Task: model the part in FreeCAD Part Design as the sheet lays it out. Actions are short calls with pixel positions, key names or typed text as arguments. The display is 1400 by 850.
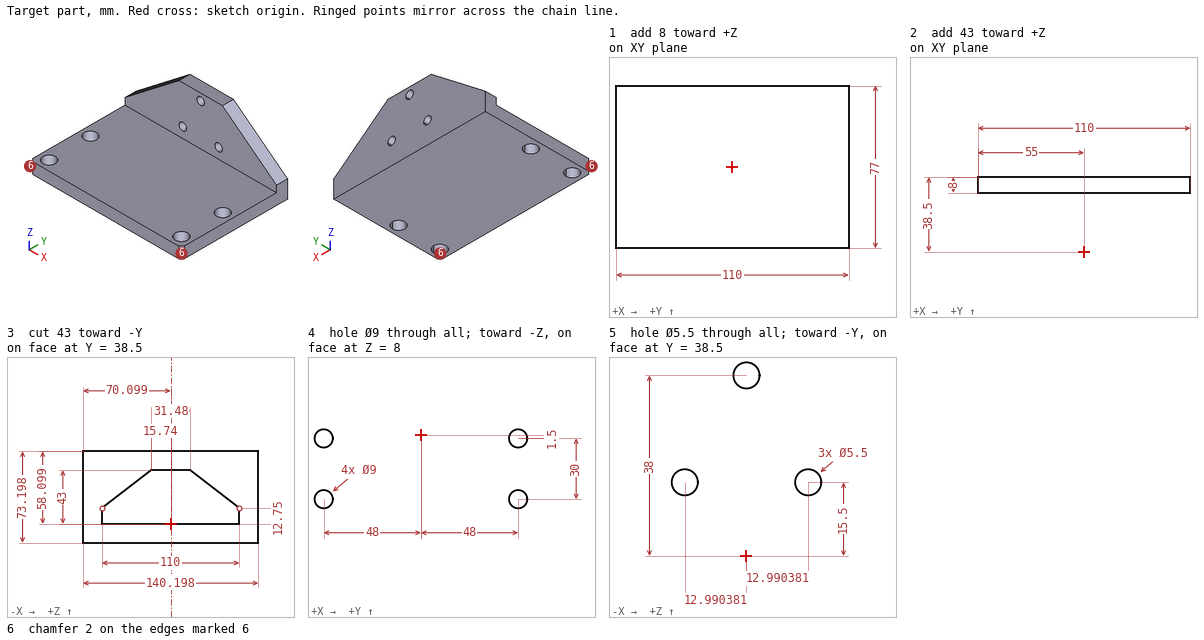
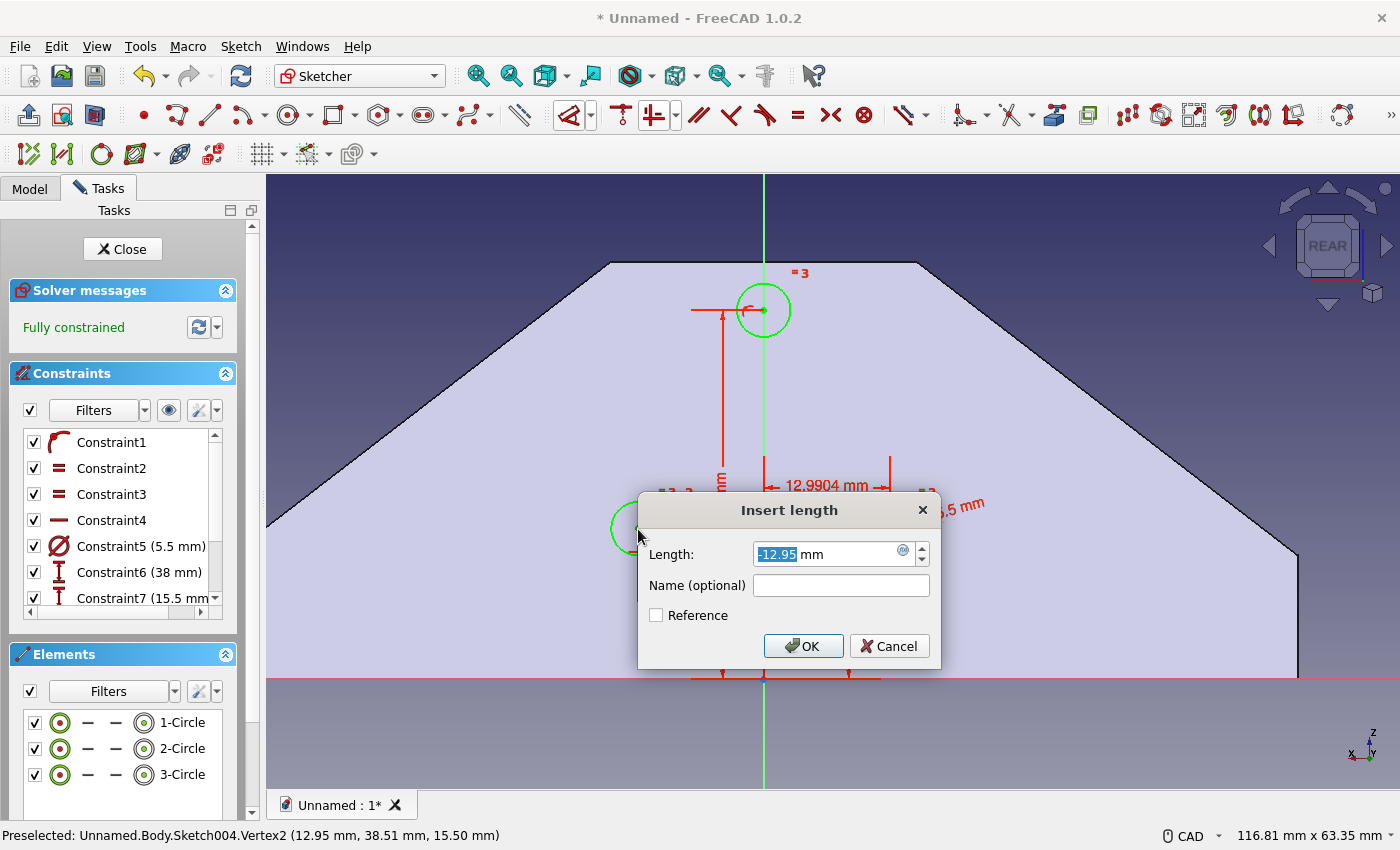
text(-12.990381)
key(Return)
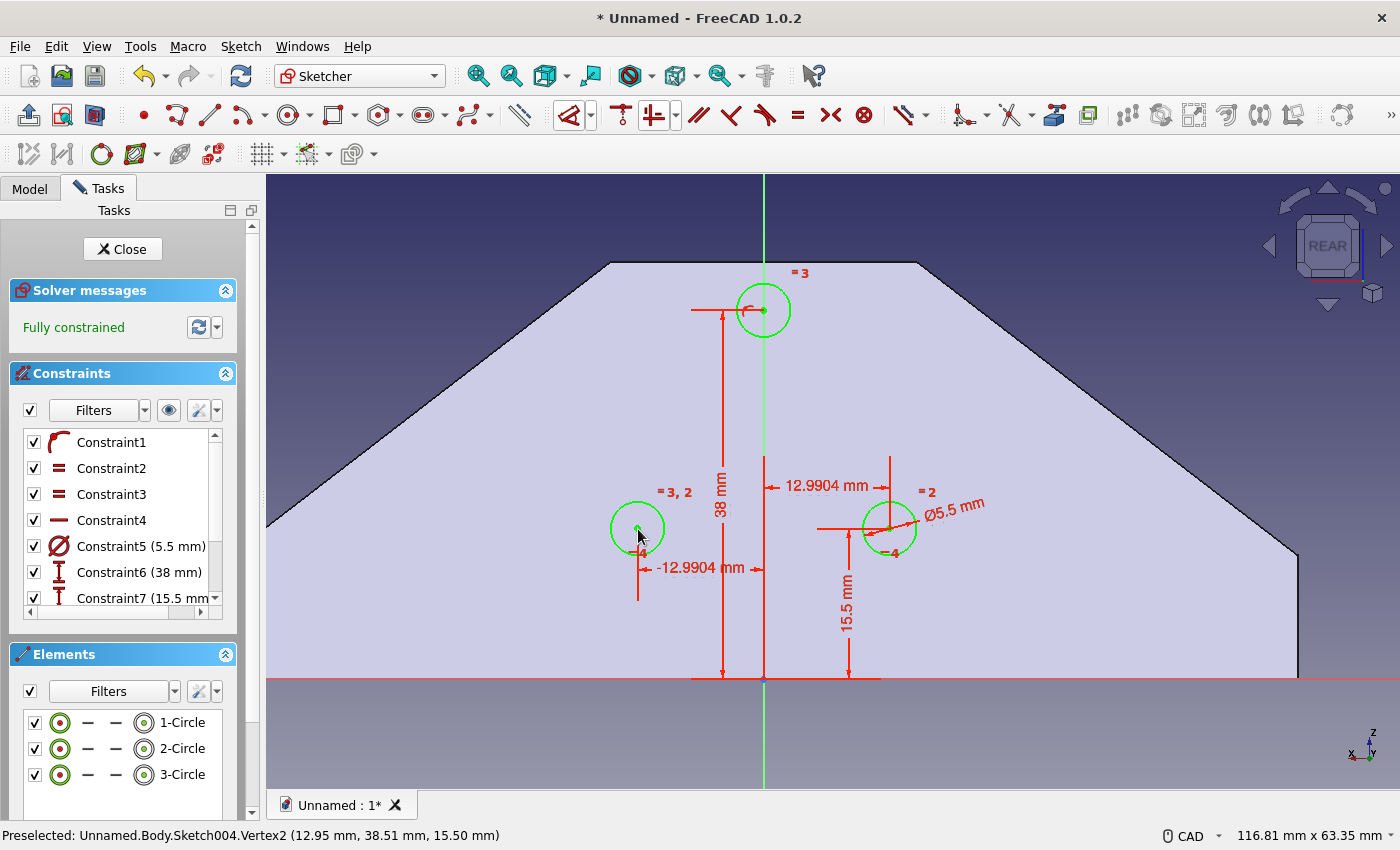
click(123, 249)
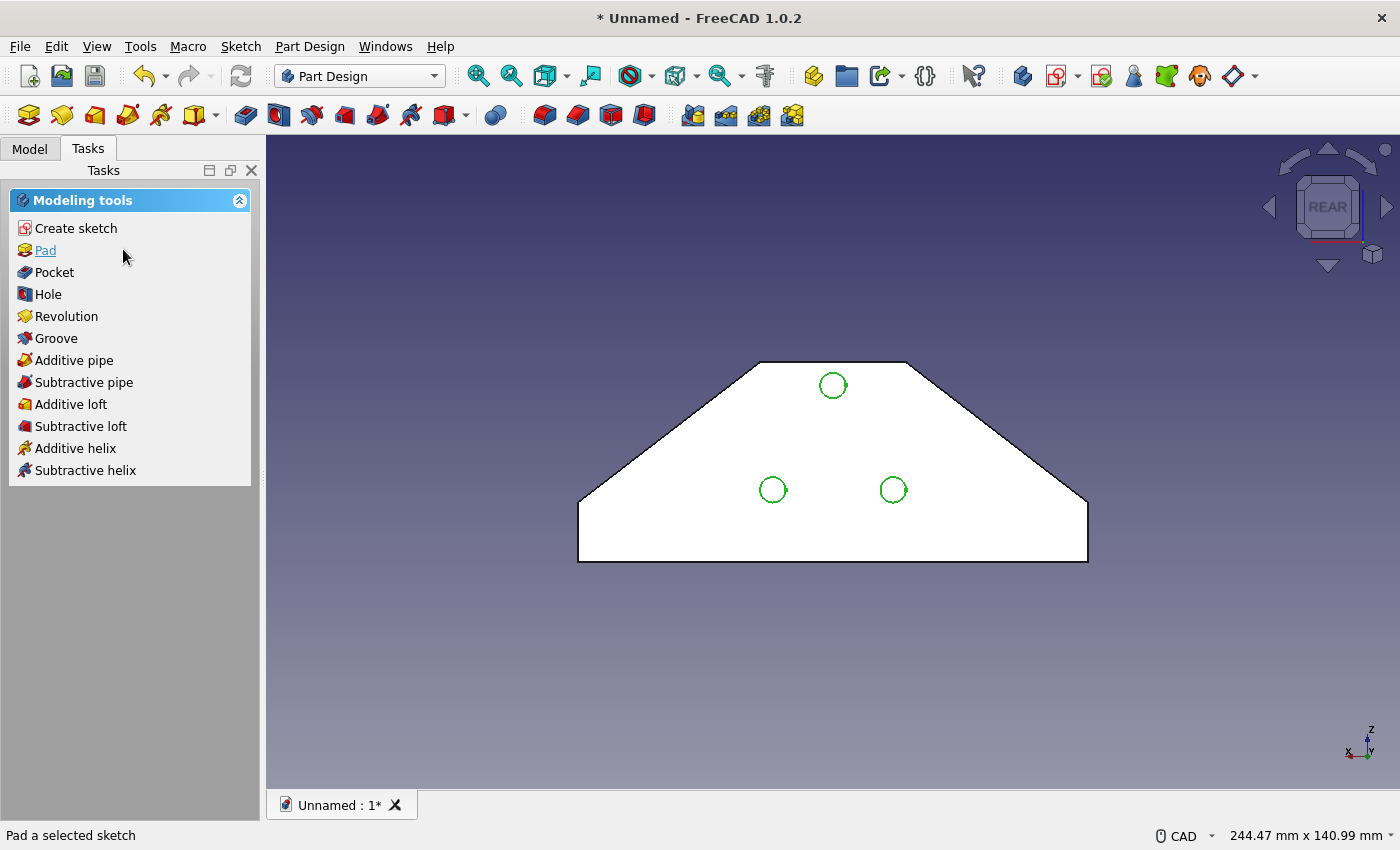
click(279, 116)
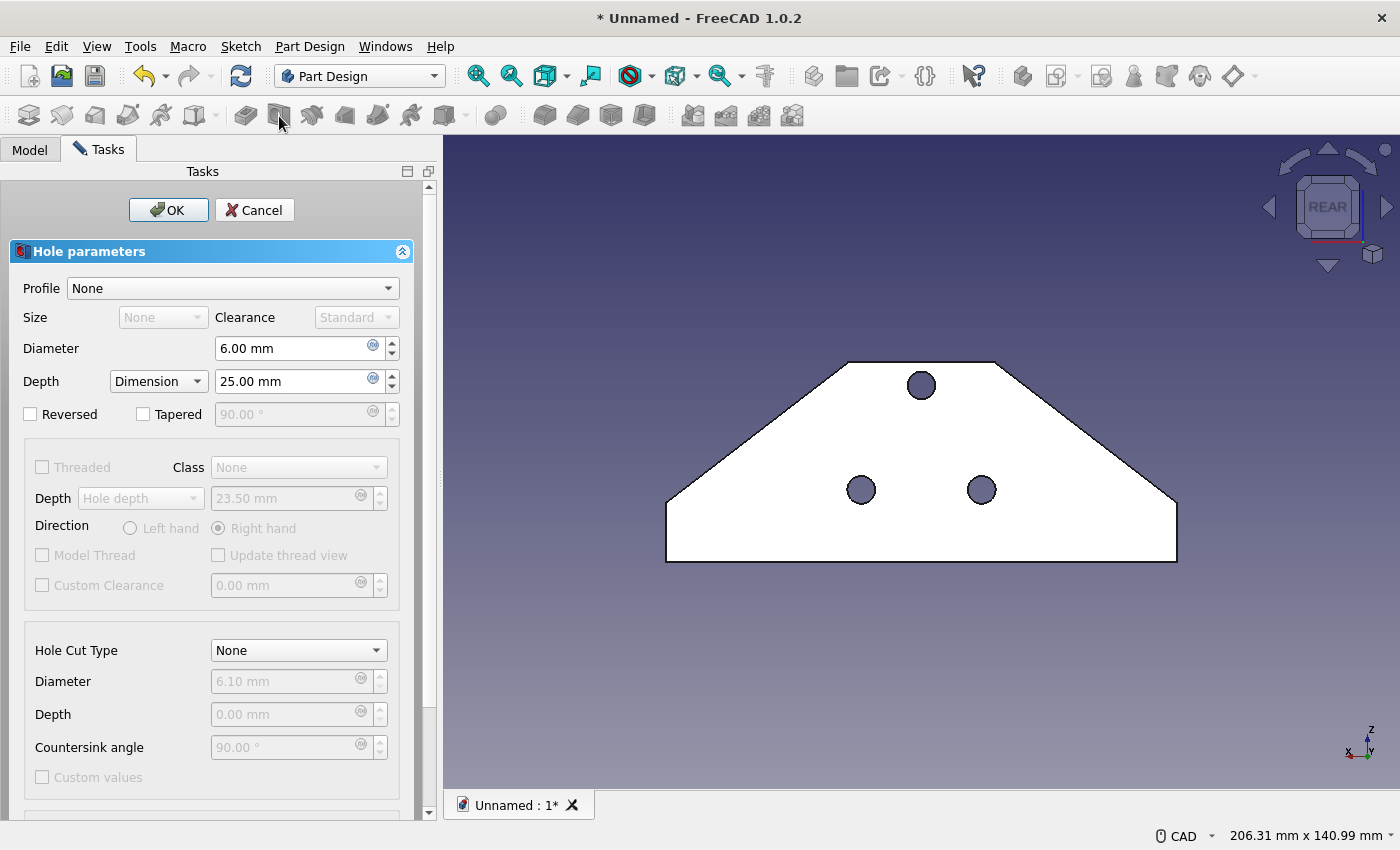
triple_click(300, 348)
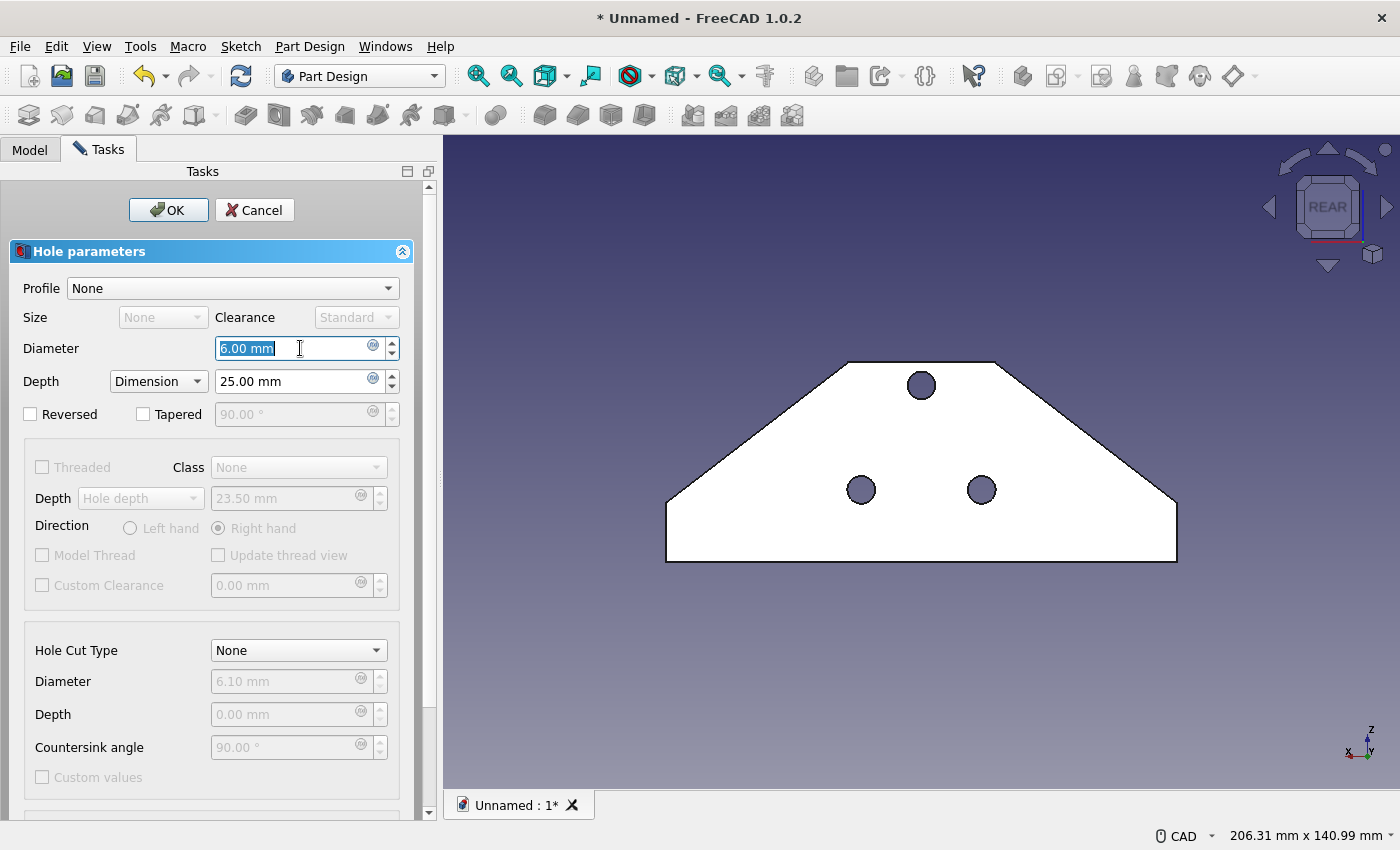
text(5.5)
key(Tab)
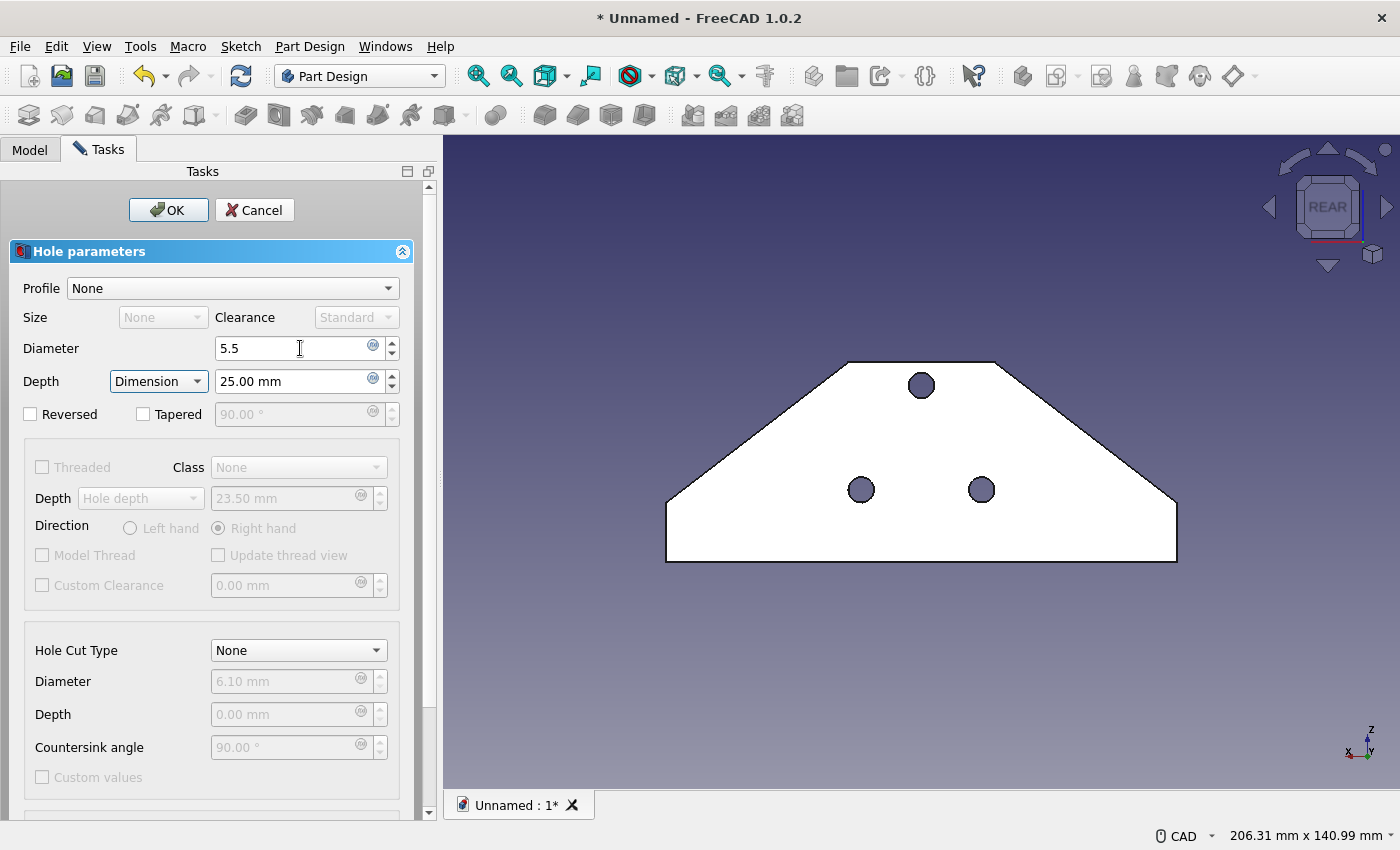
click(160, 382)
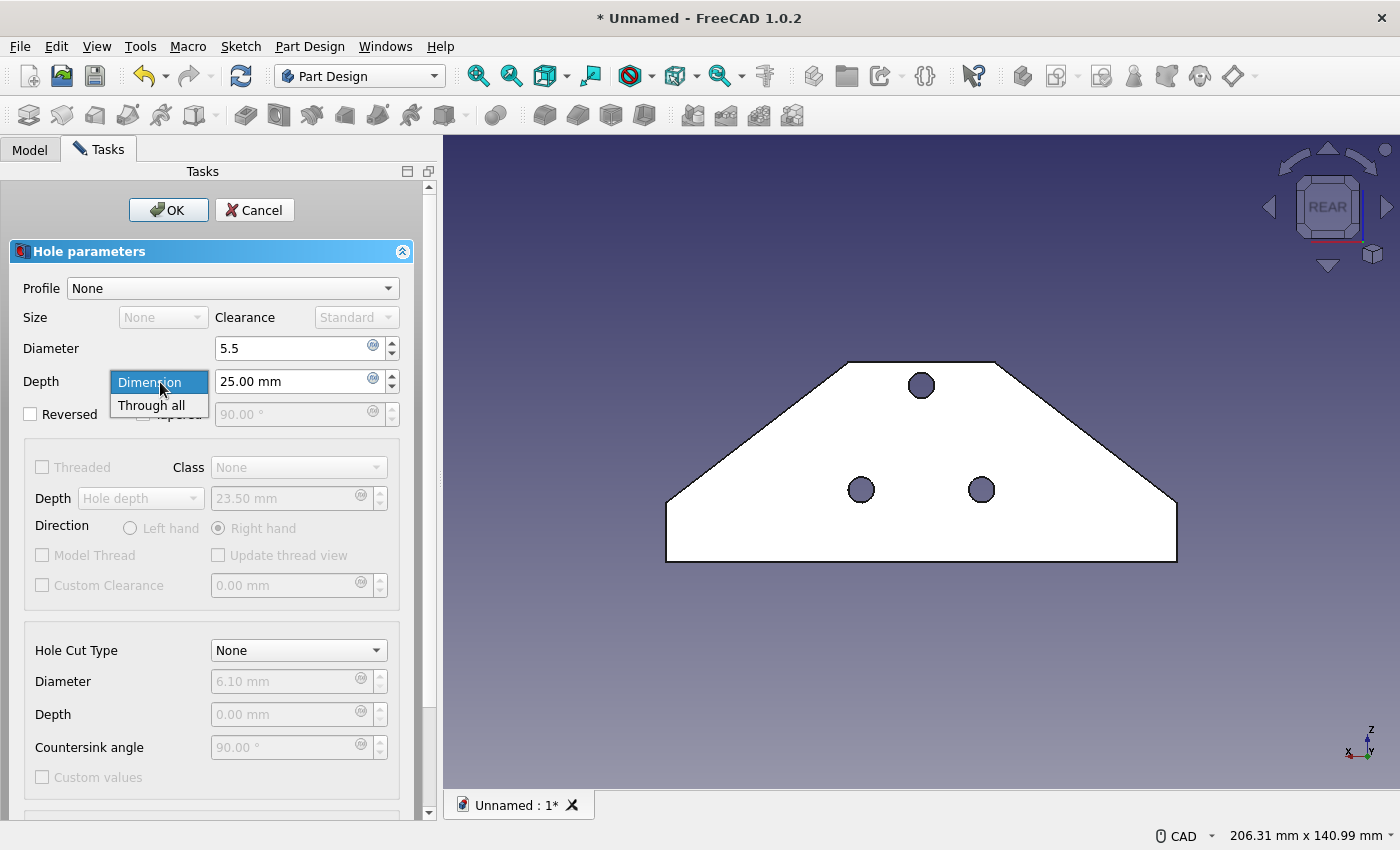
click(158, 406)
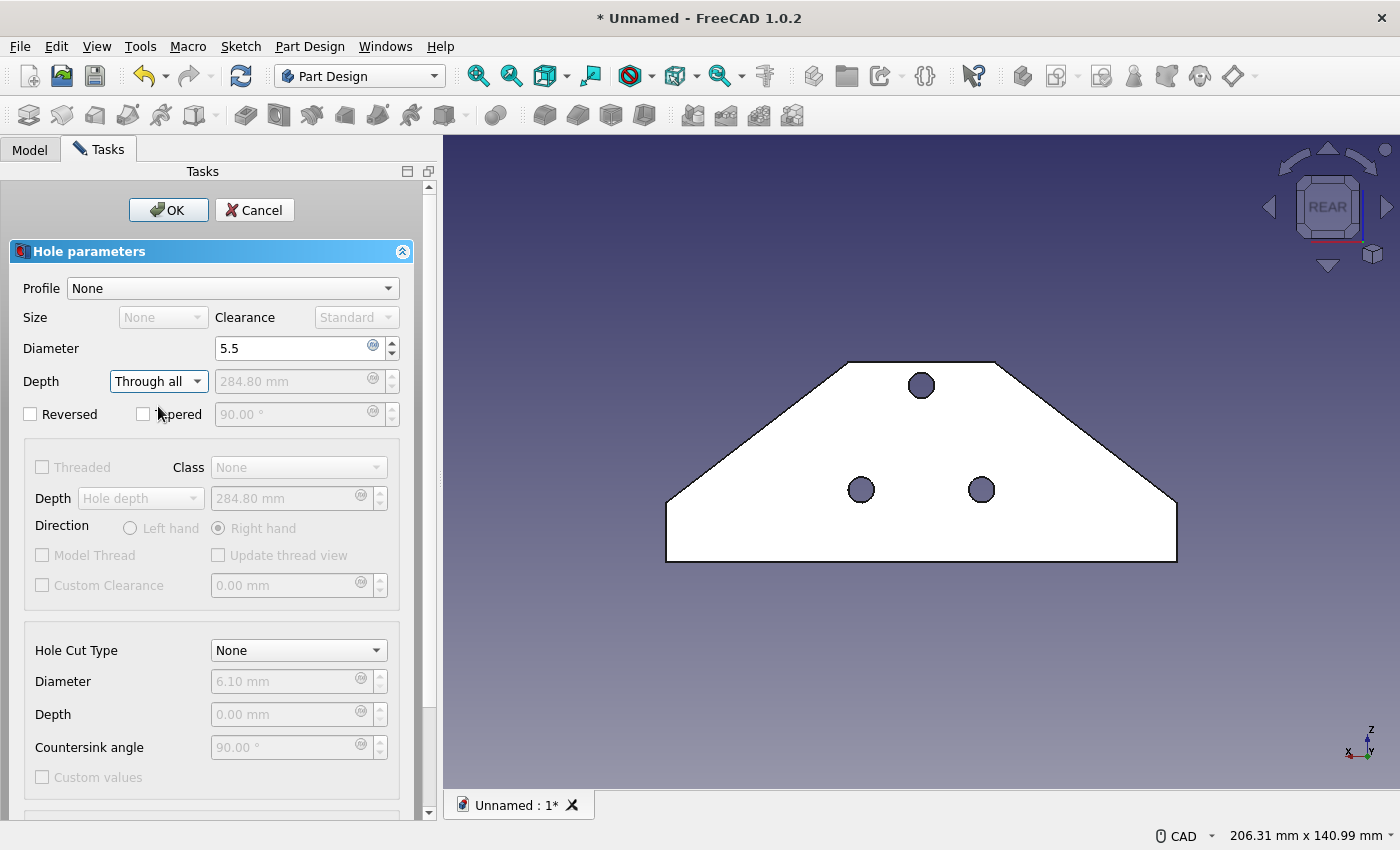
click(169, 210)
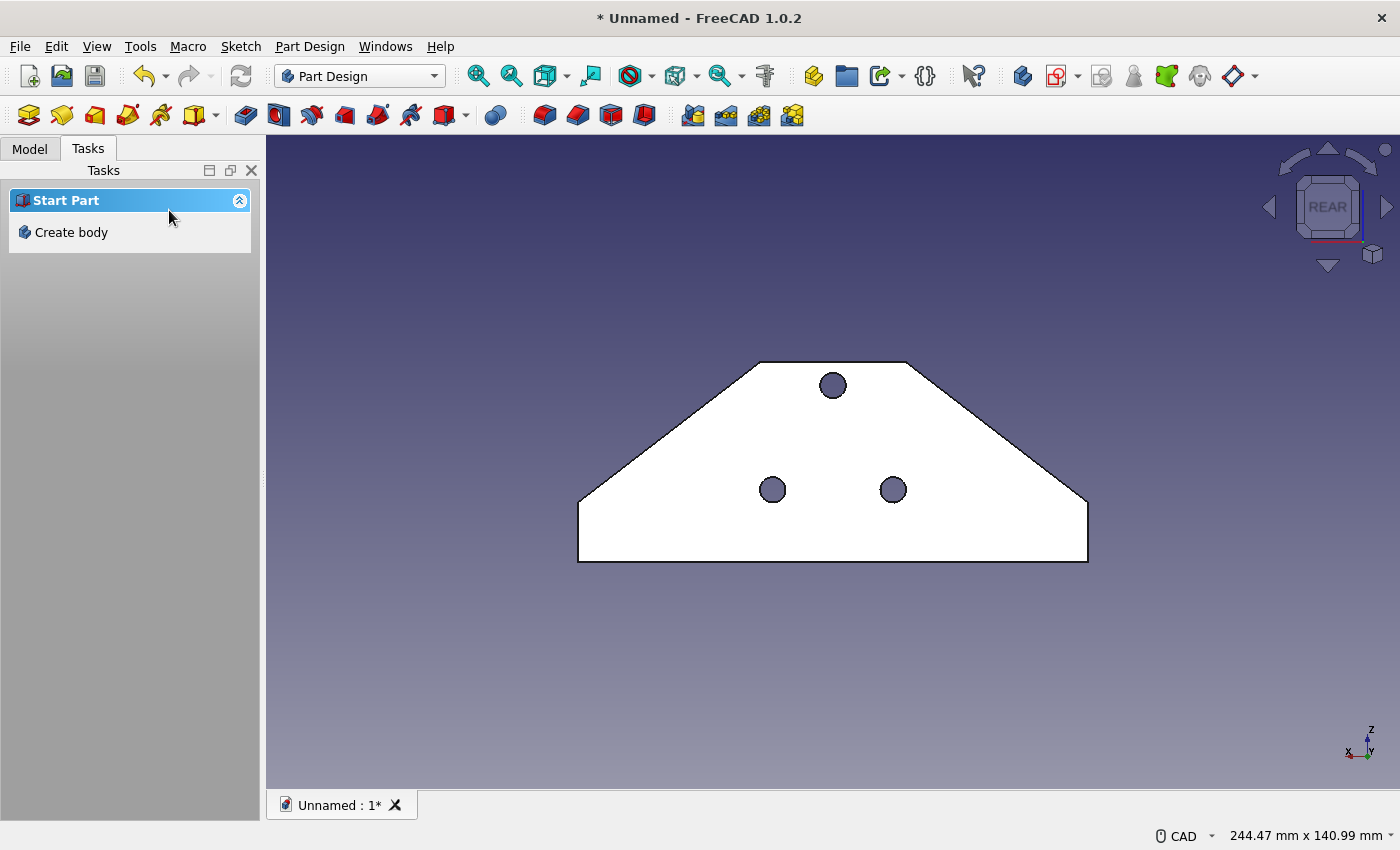
key(v)
key(f)